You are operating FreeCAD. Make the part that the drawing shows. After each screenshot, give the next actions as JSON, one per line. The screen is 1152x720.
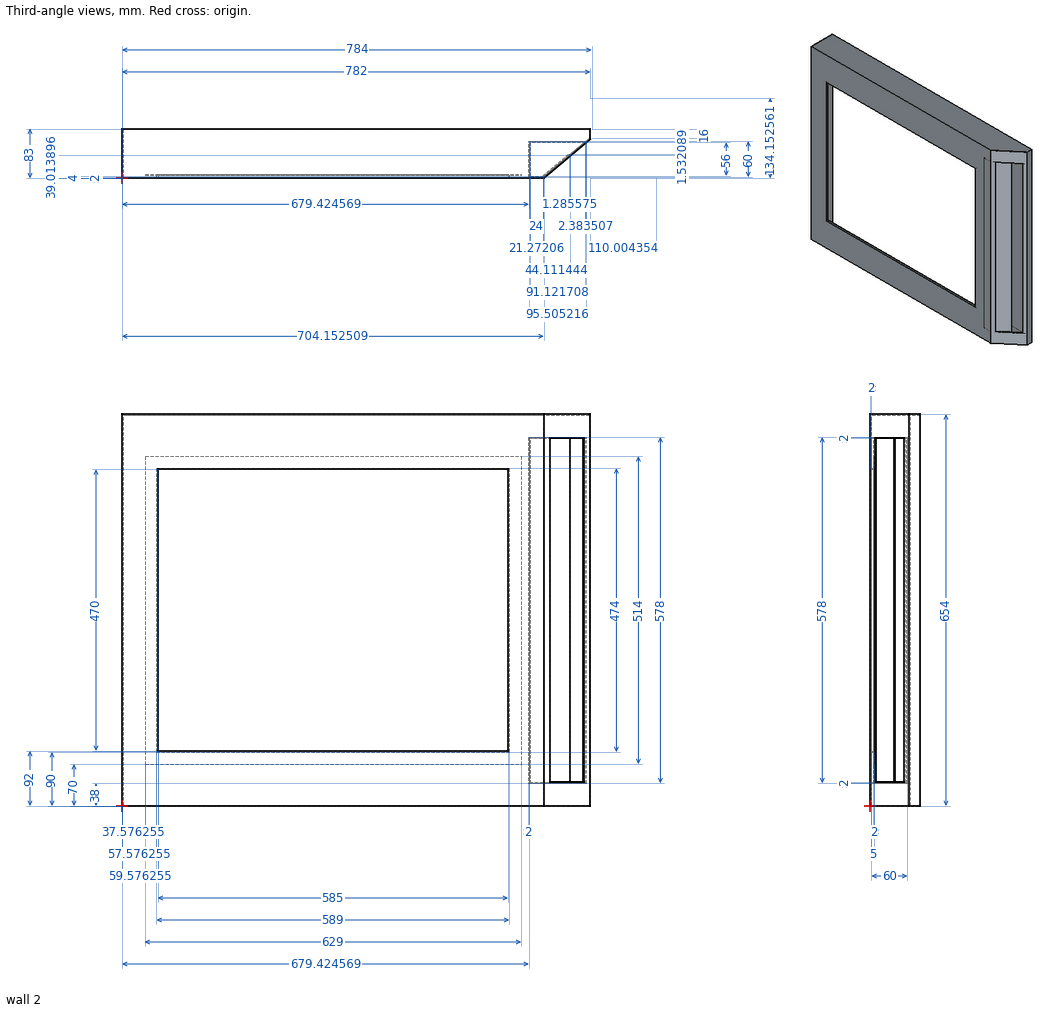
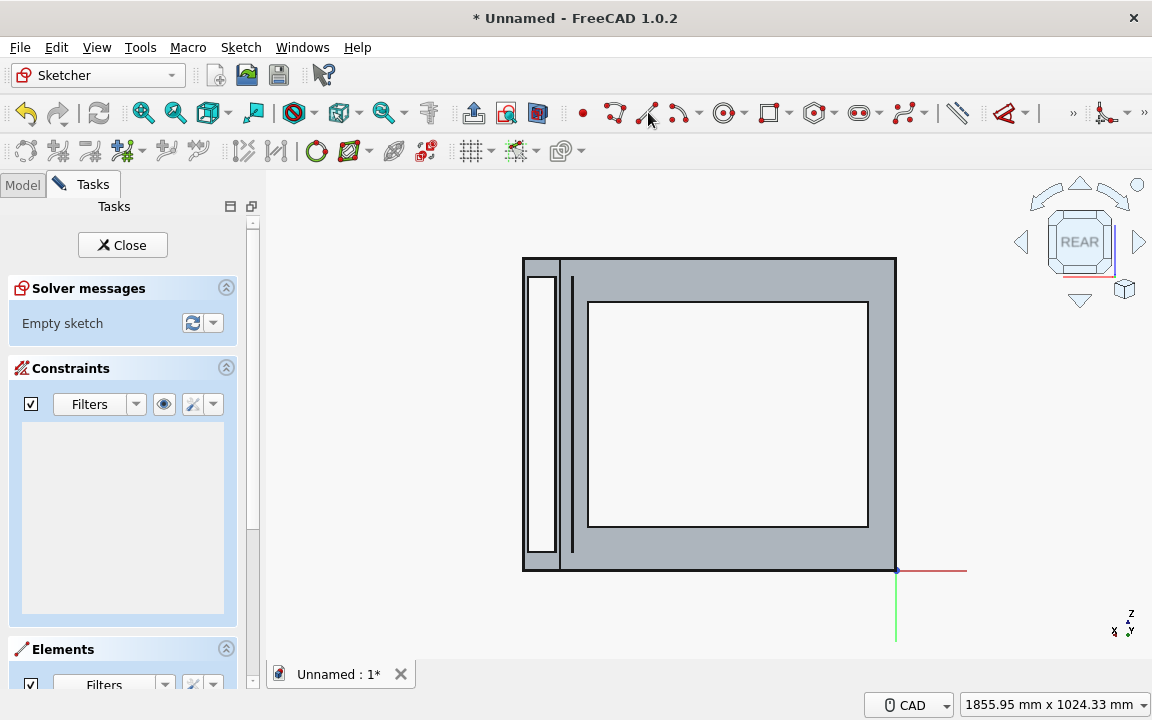
{"action": "key", "text": "g r"}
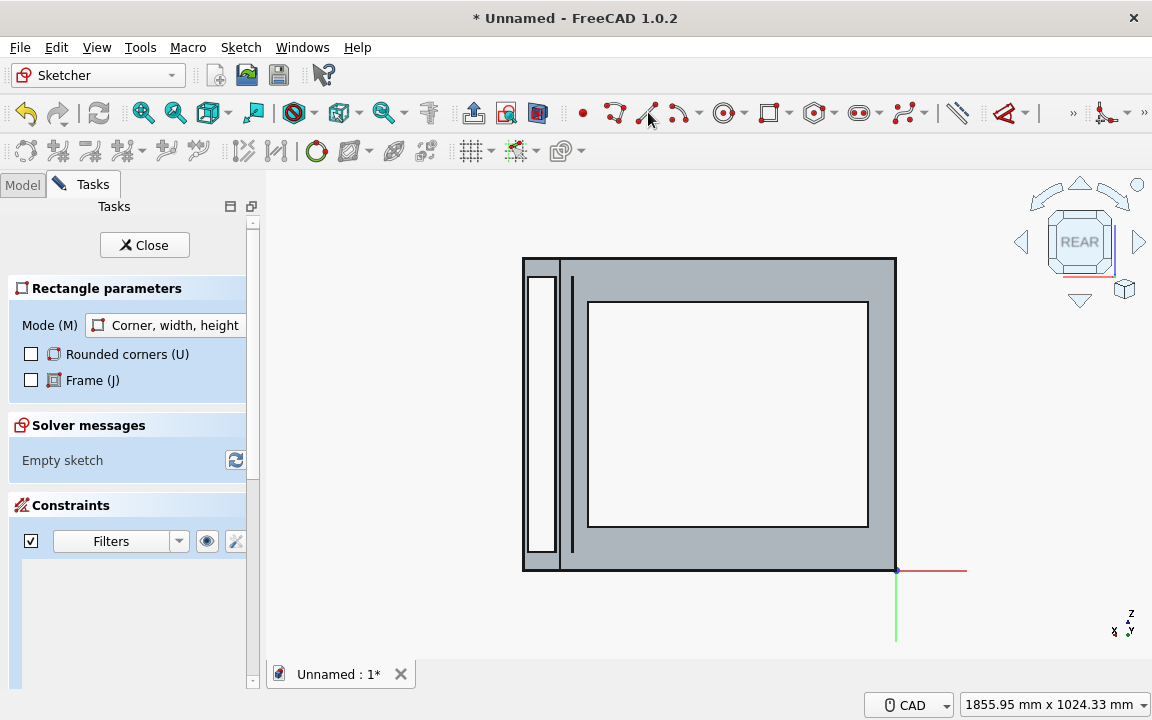
{"action": "left_click", "coordinate": [587, 301]}
{"action": "left_click", "coordinate": [869, 528]}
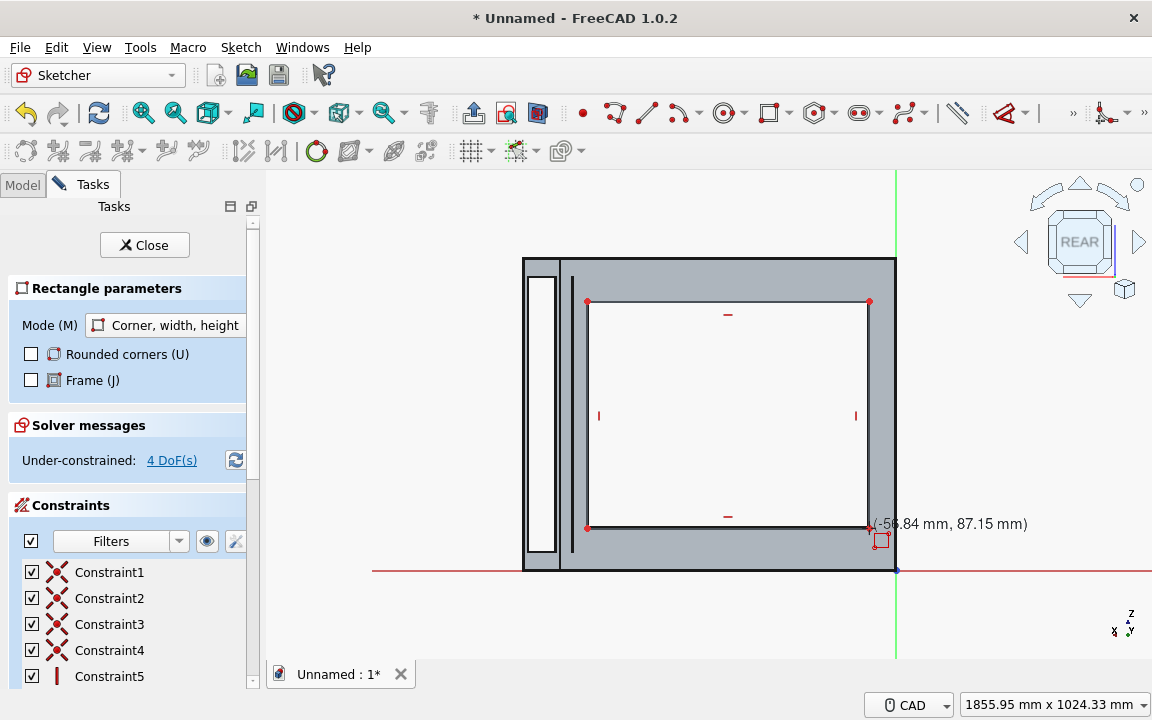
{"action": "scroll", "coordinate": [588, 302], "scroll_direction": "up", "scroll_amount": 15}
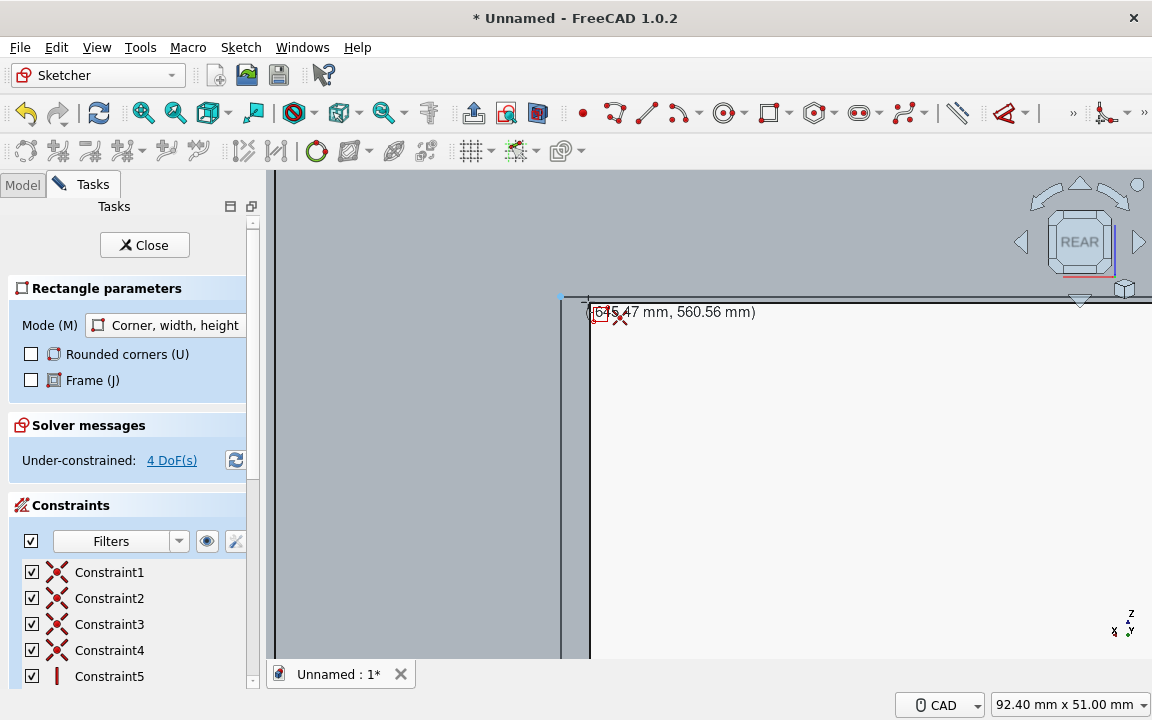
{"action": "left_click", "coordinate": [590, 303]}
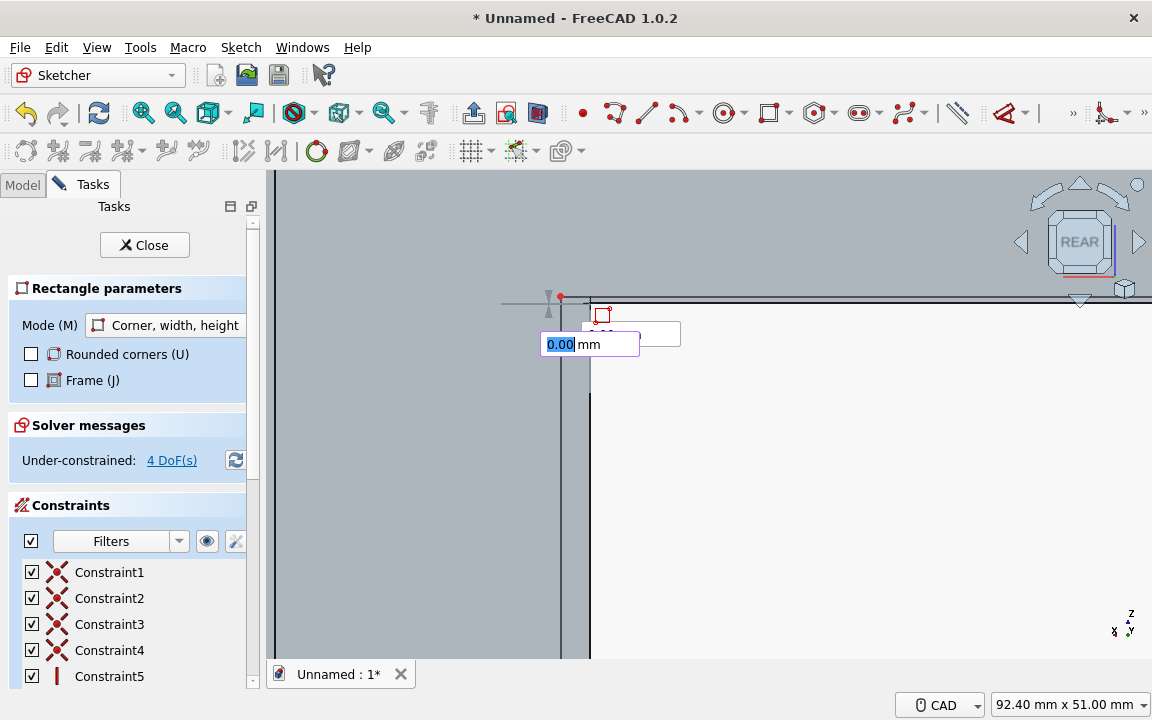
{"action": "scroll", "coordinate": [444, 248], "scroll_direction": "down", "scroll_amount": 14}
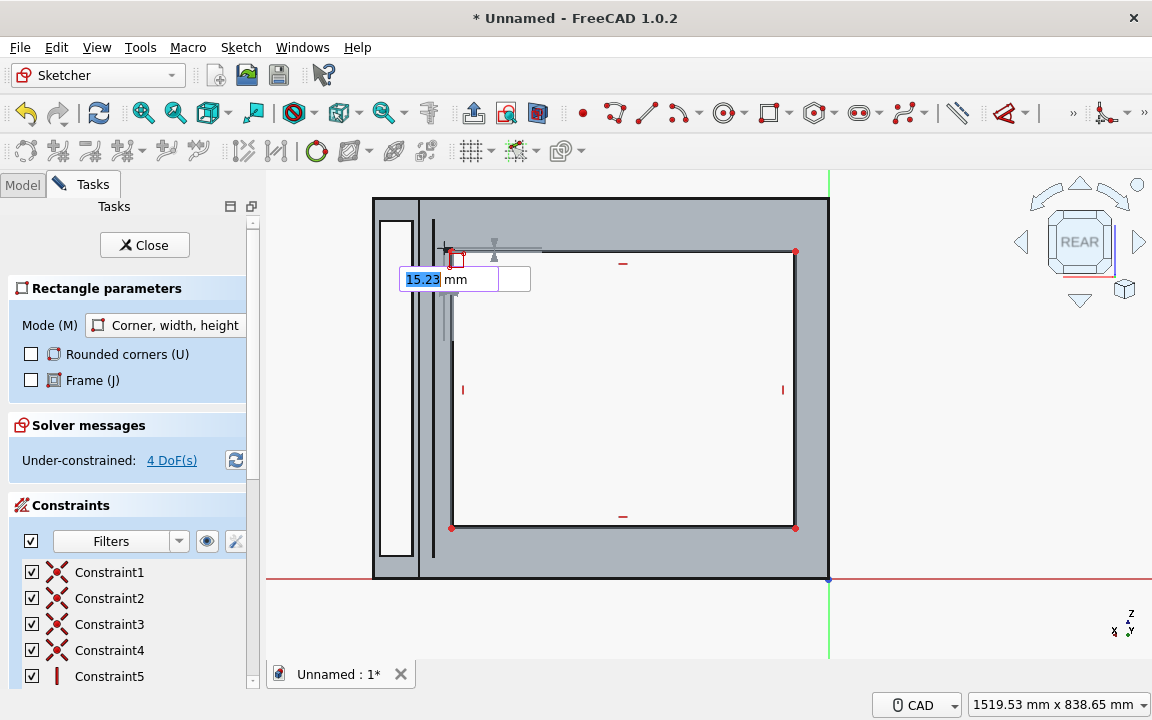
{"action": "scroll", "coordinate": [794, 526], "scroll_direction": "up", "scroll_amount": 14}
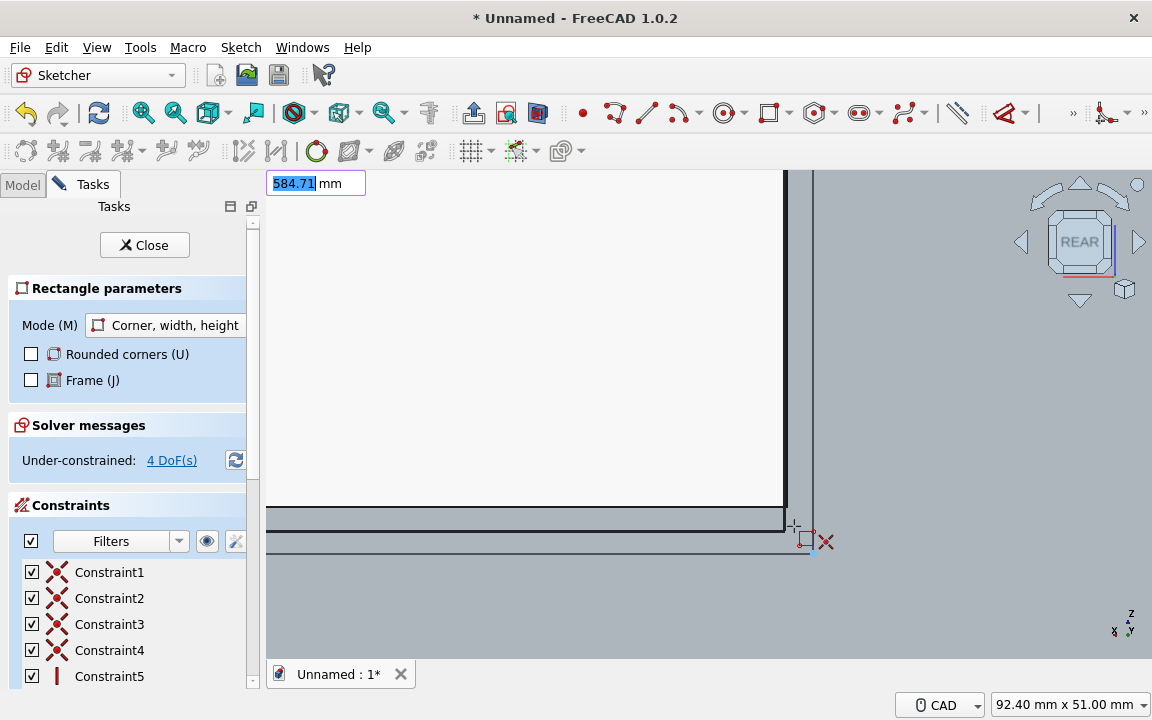
{"action": "left_click", "coordinate": [787, 507]}
{"action": "key", "text": "Escape"}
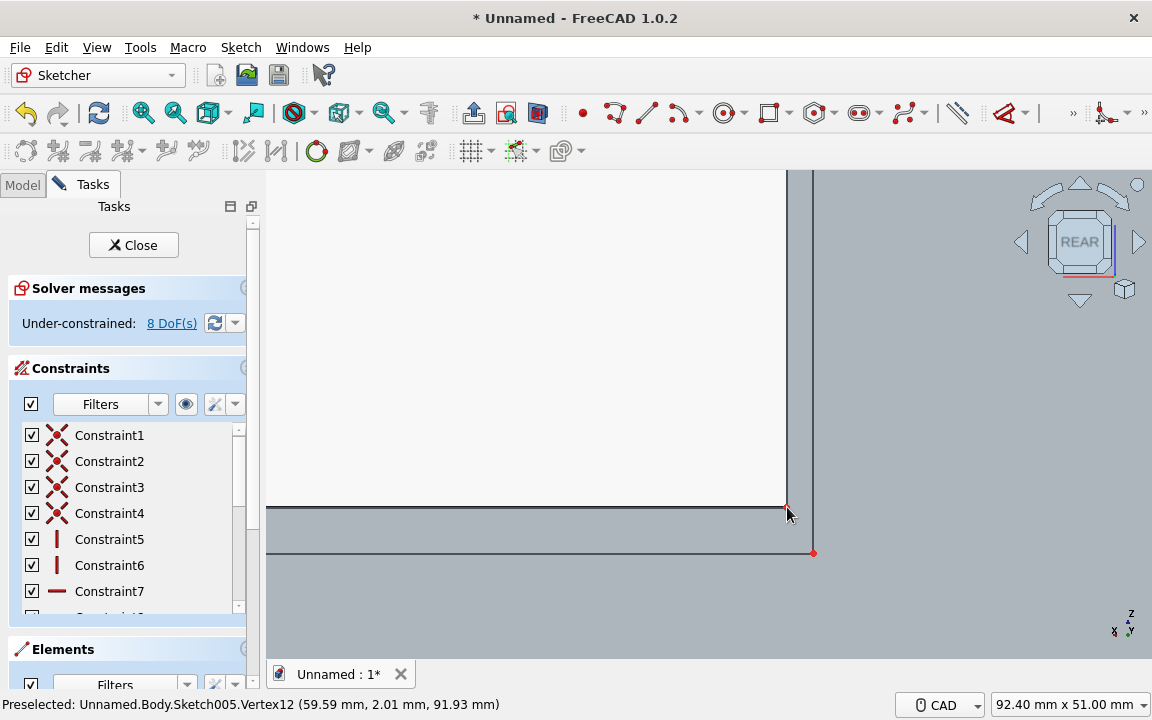
{"action": "key", "text": "d"}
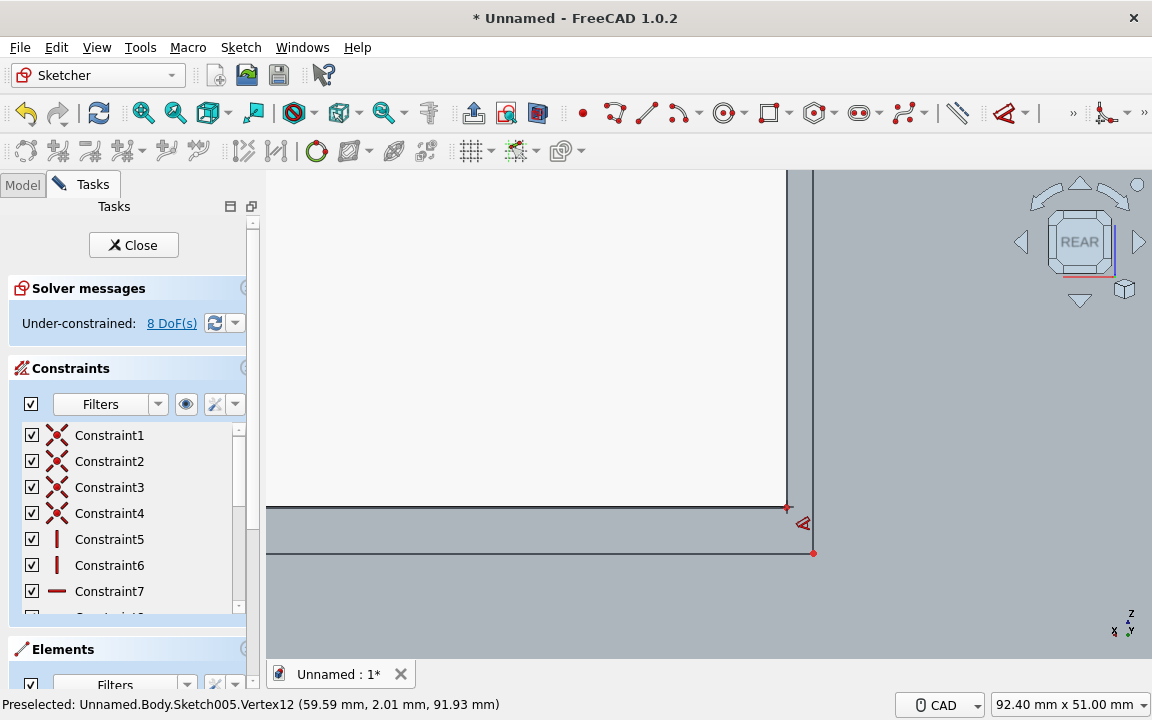
{"action": "scroll", "coordinate": [795, 526], "scroll_direction": "down", "scroll_amount": 14}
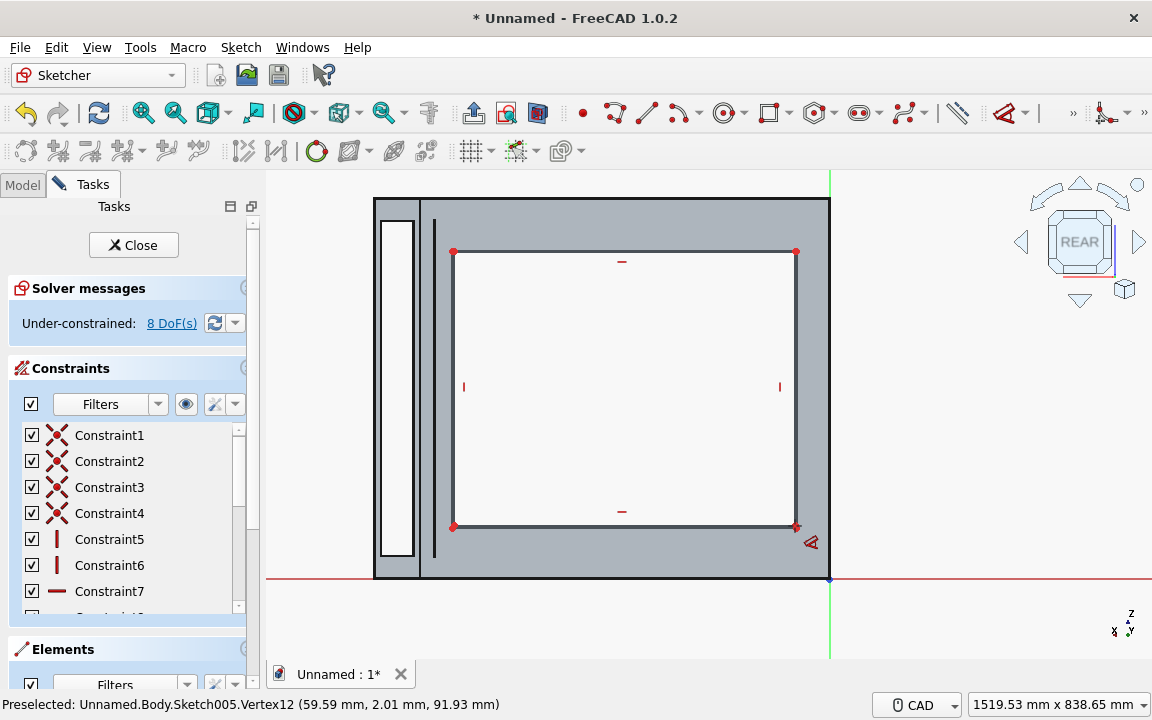
{"action": "scroll", "coordinate": [452, 334], "scroll_direction": "up", "scroll_amount": 11}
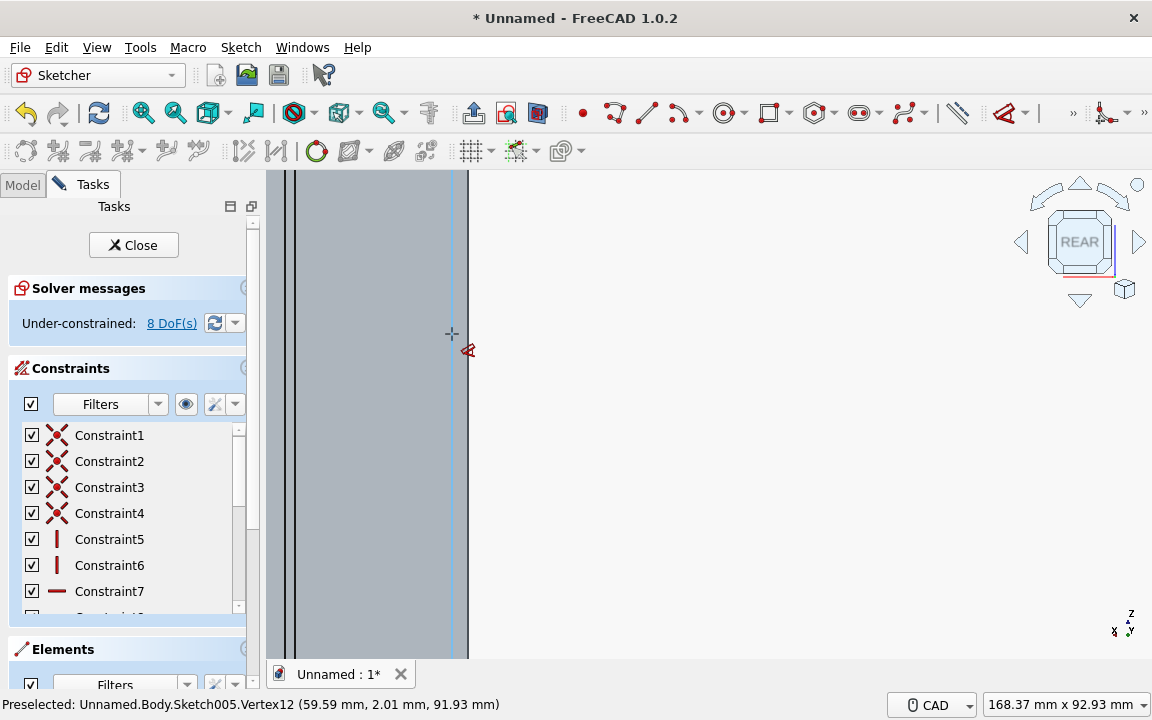
{"action": "left_click", "coordinate": [452, 334]}
{"action": "left_click", "coordinate": [418, 414]}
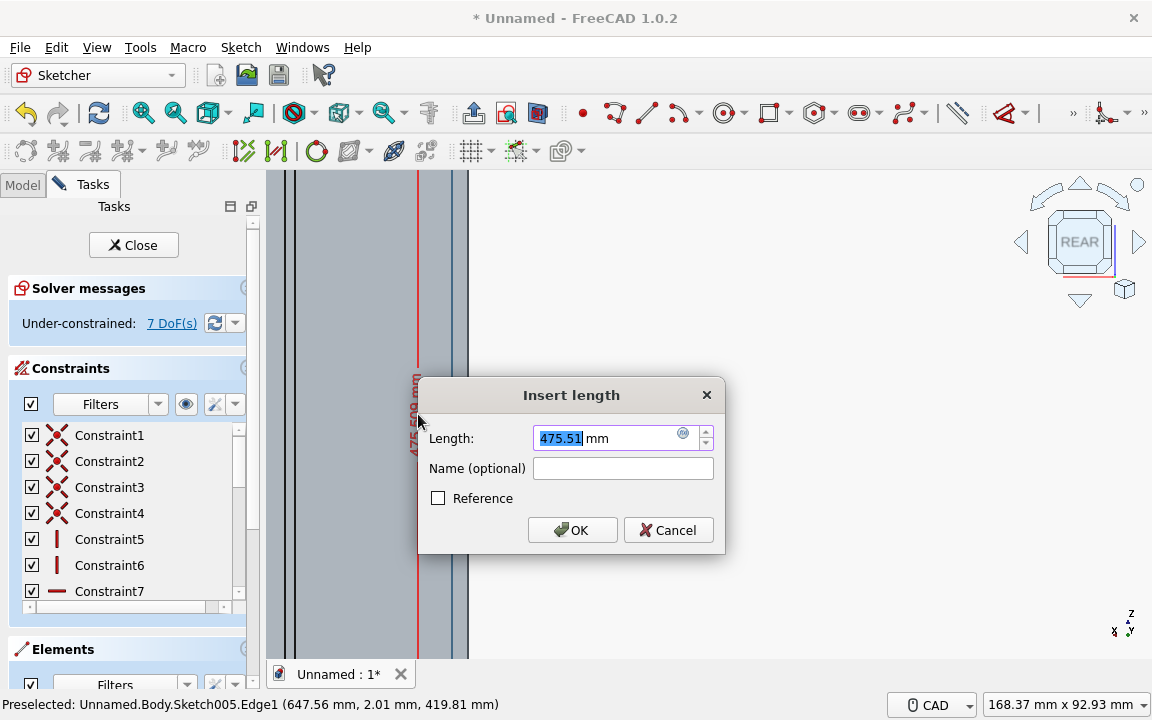
{"action": "type", "text": "474"}
{"action": "key", "text": "Return"}